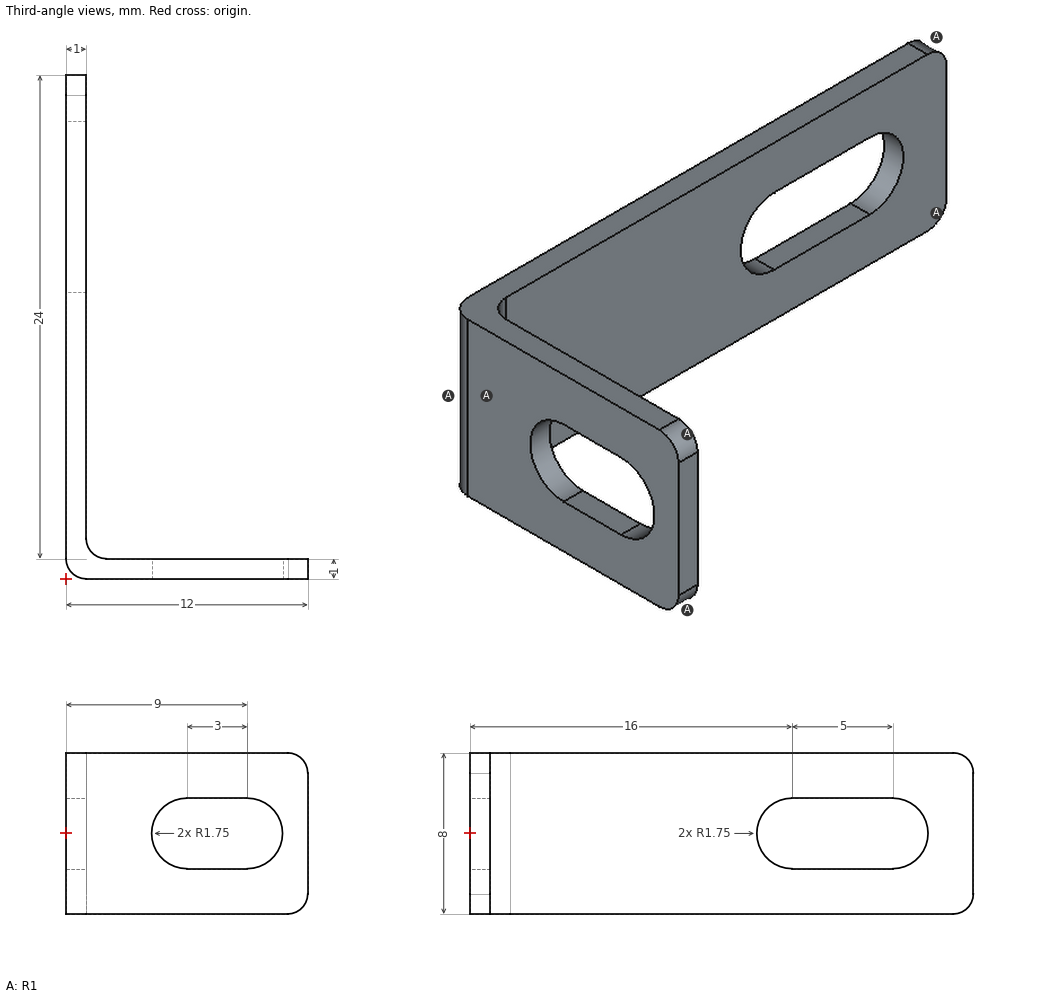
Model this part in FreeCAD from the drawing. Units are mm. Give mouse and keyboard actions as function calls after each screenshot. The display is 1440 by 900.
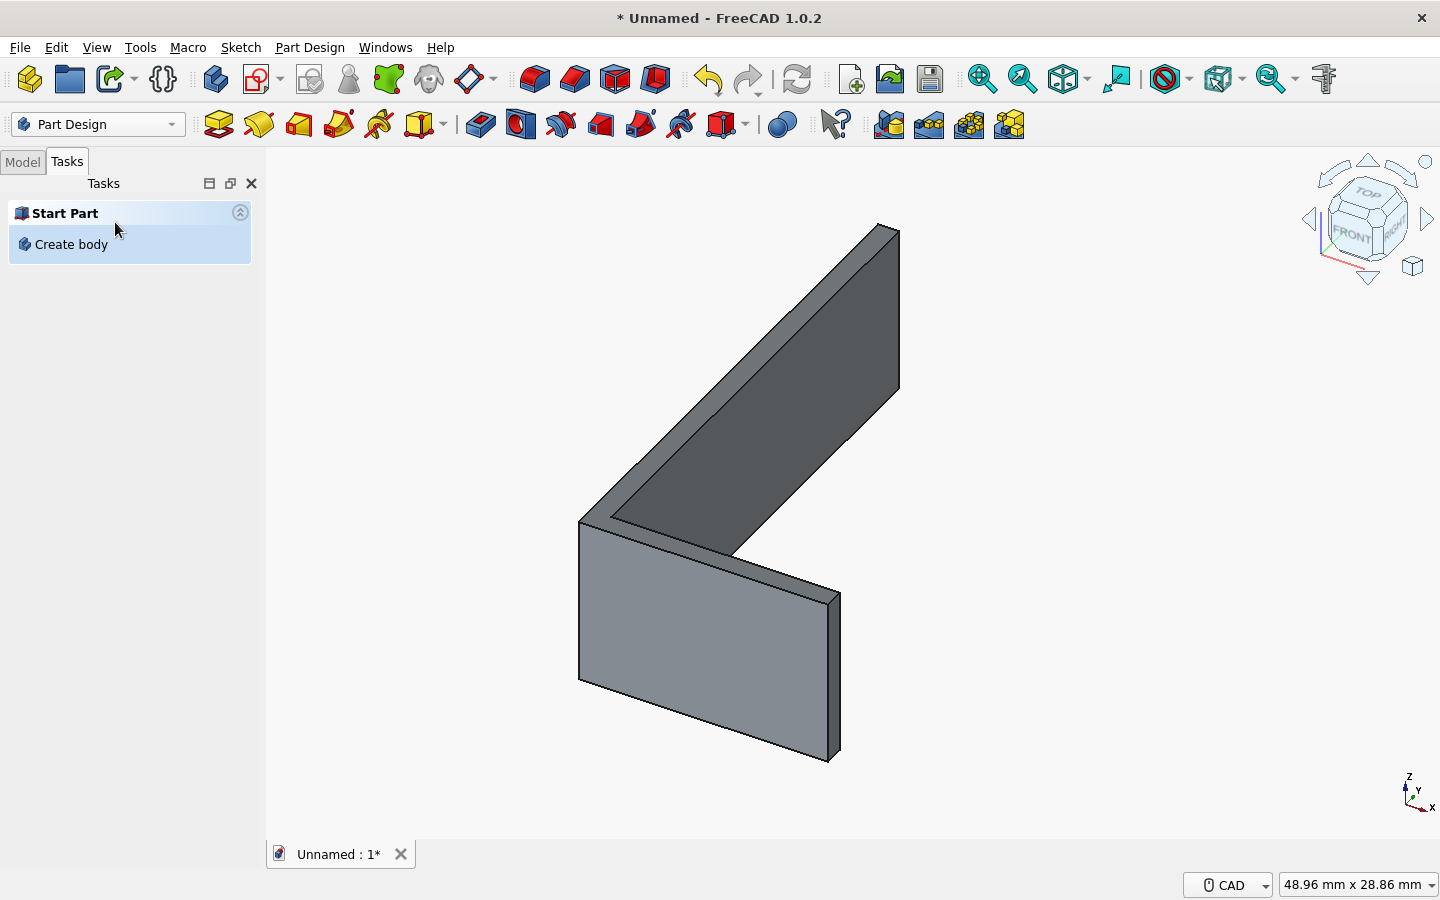
key(4)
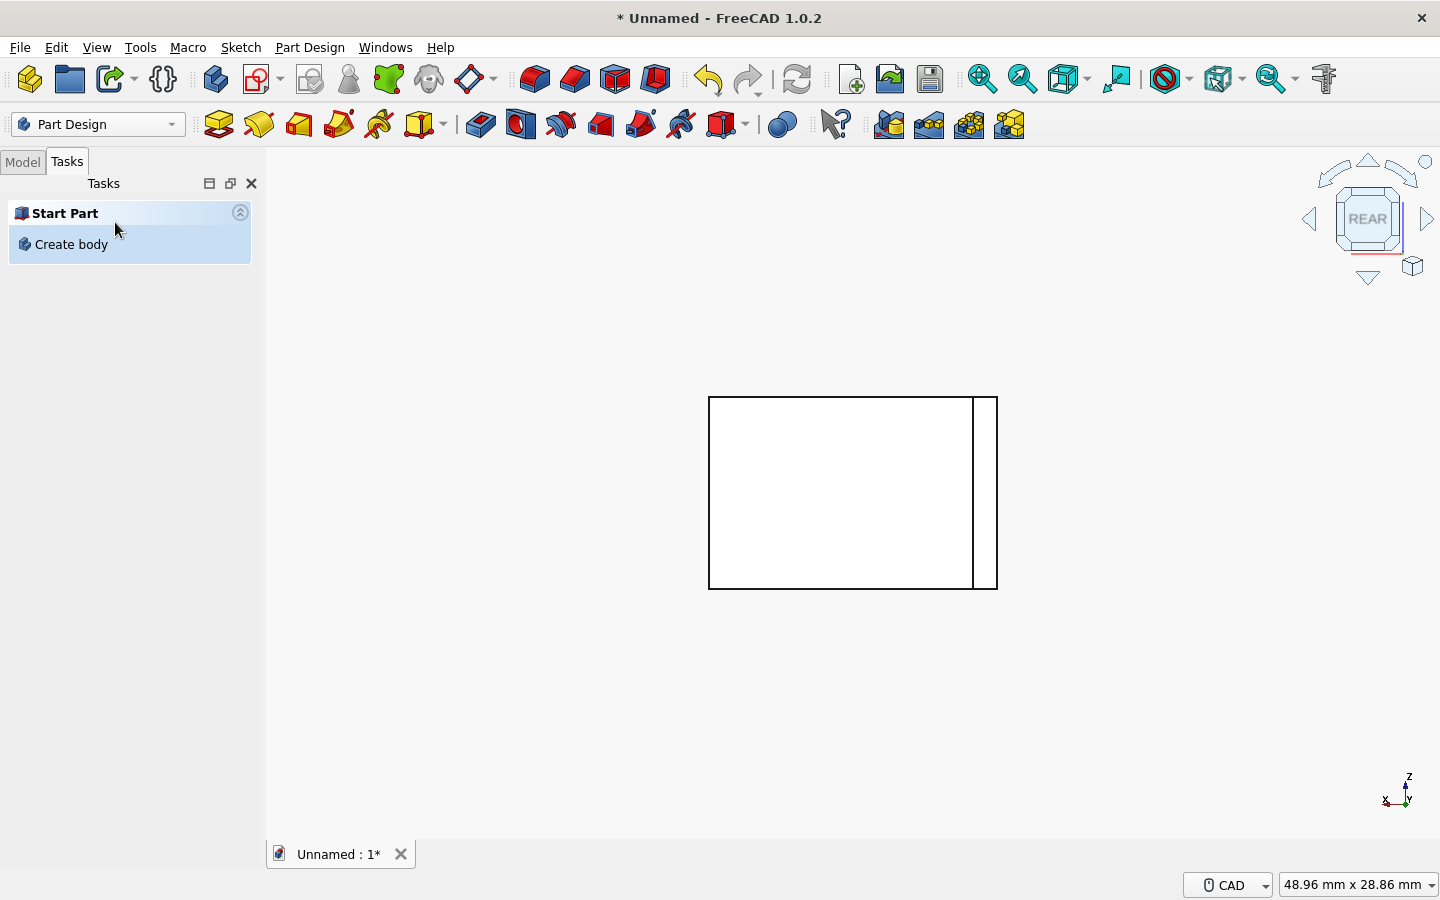
key(v)
key(f)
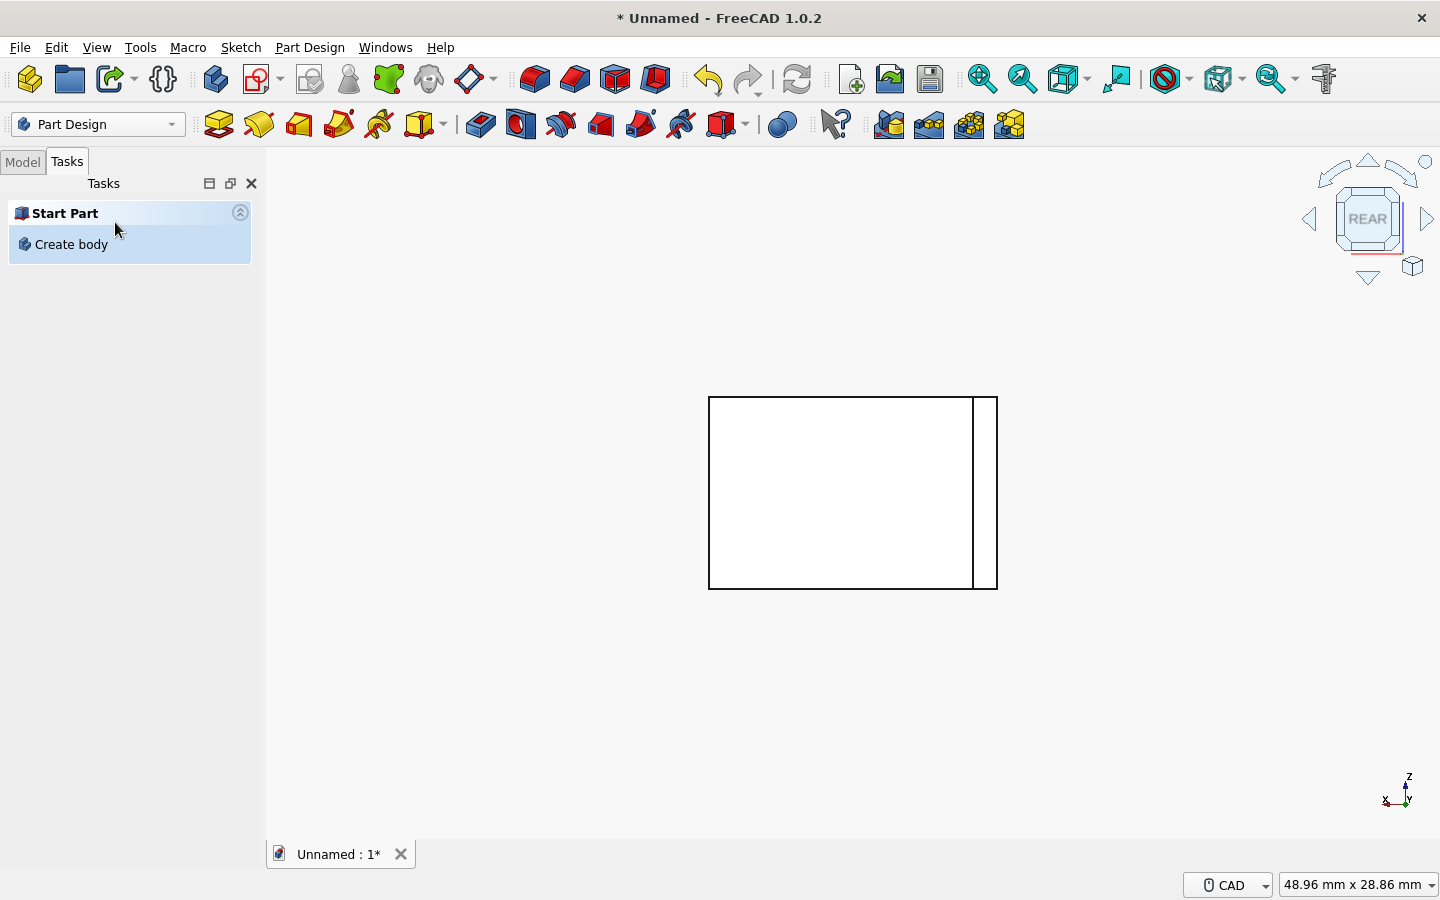
click(841, 492)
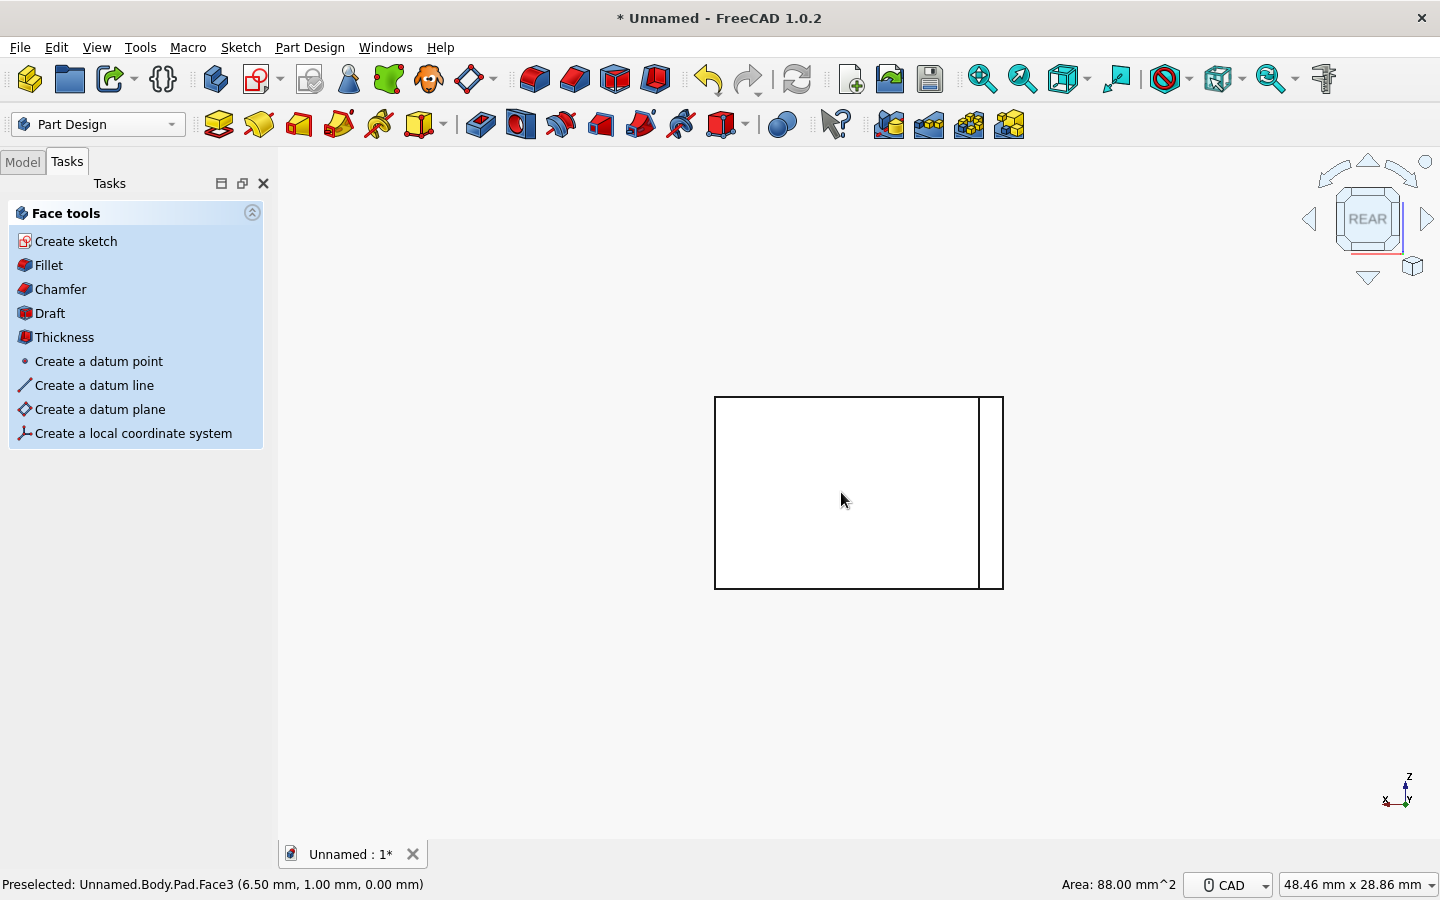
click(256, 80)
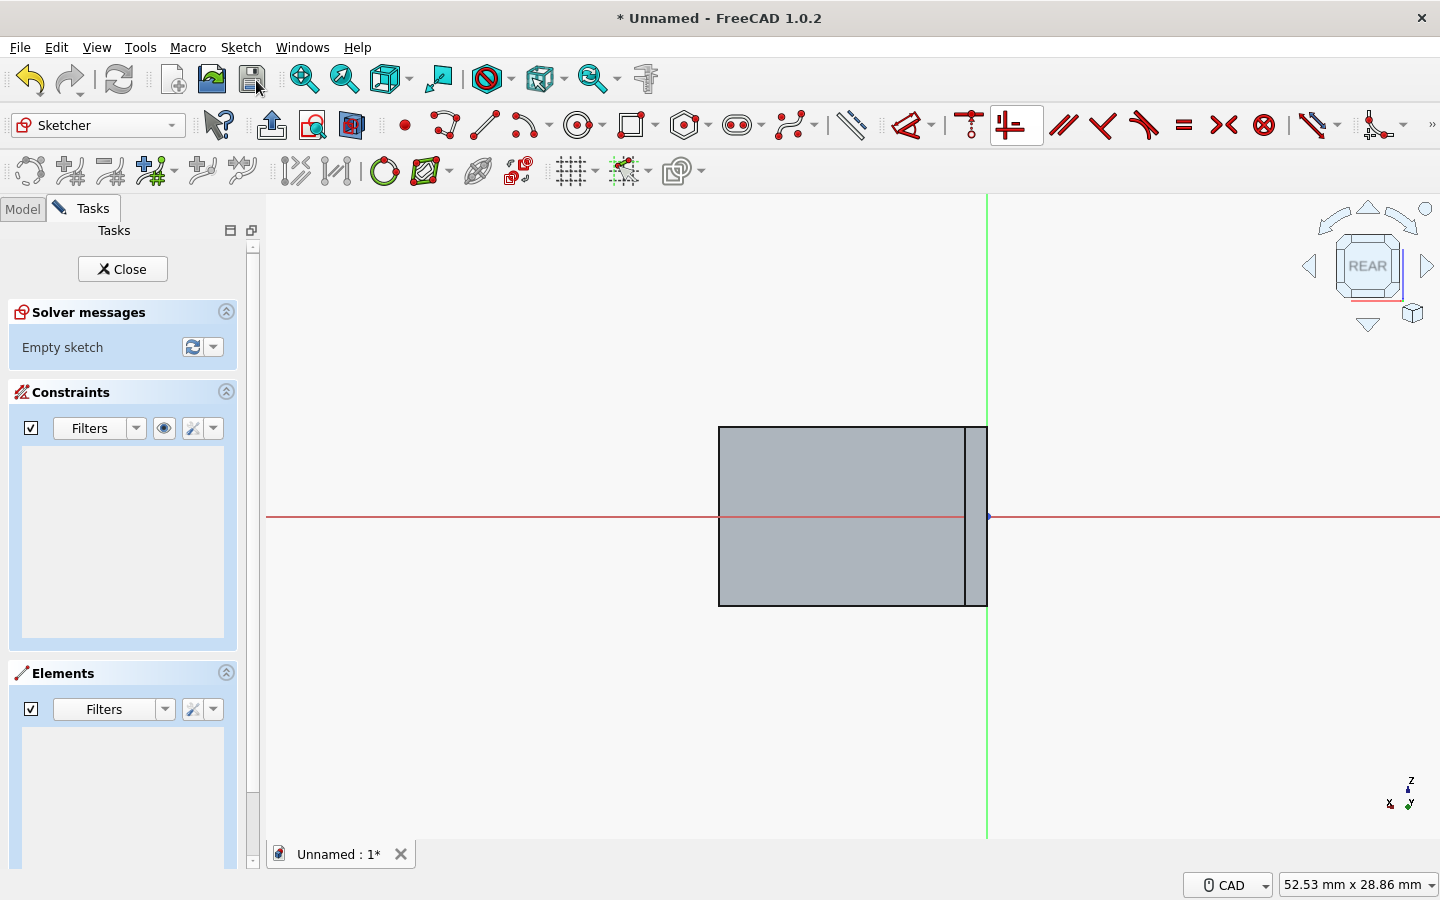
scroll(915, 517, up, 5)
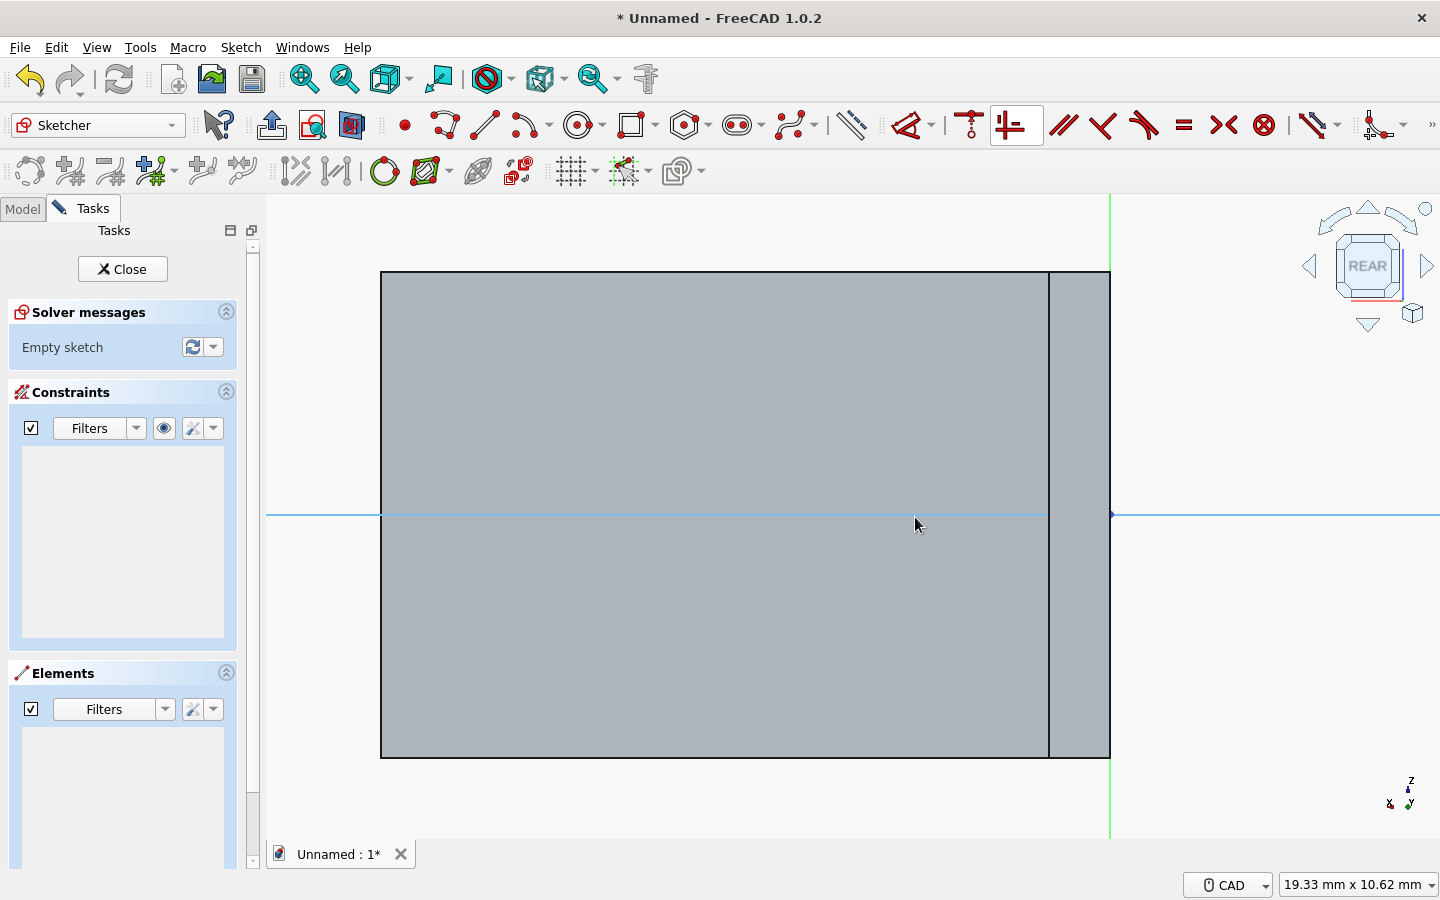
key(g)
key(s)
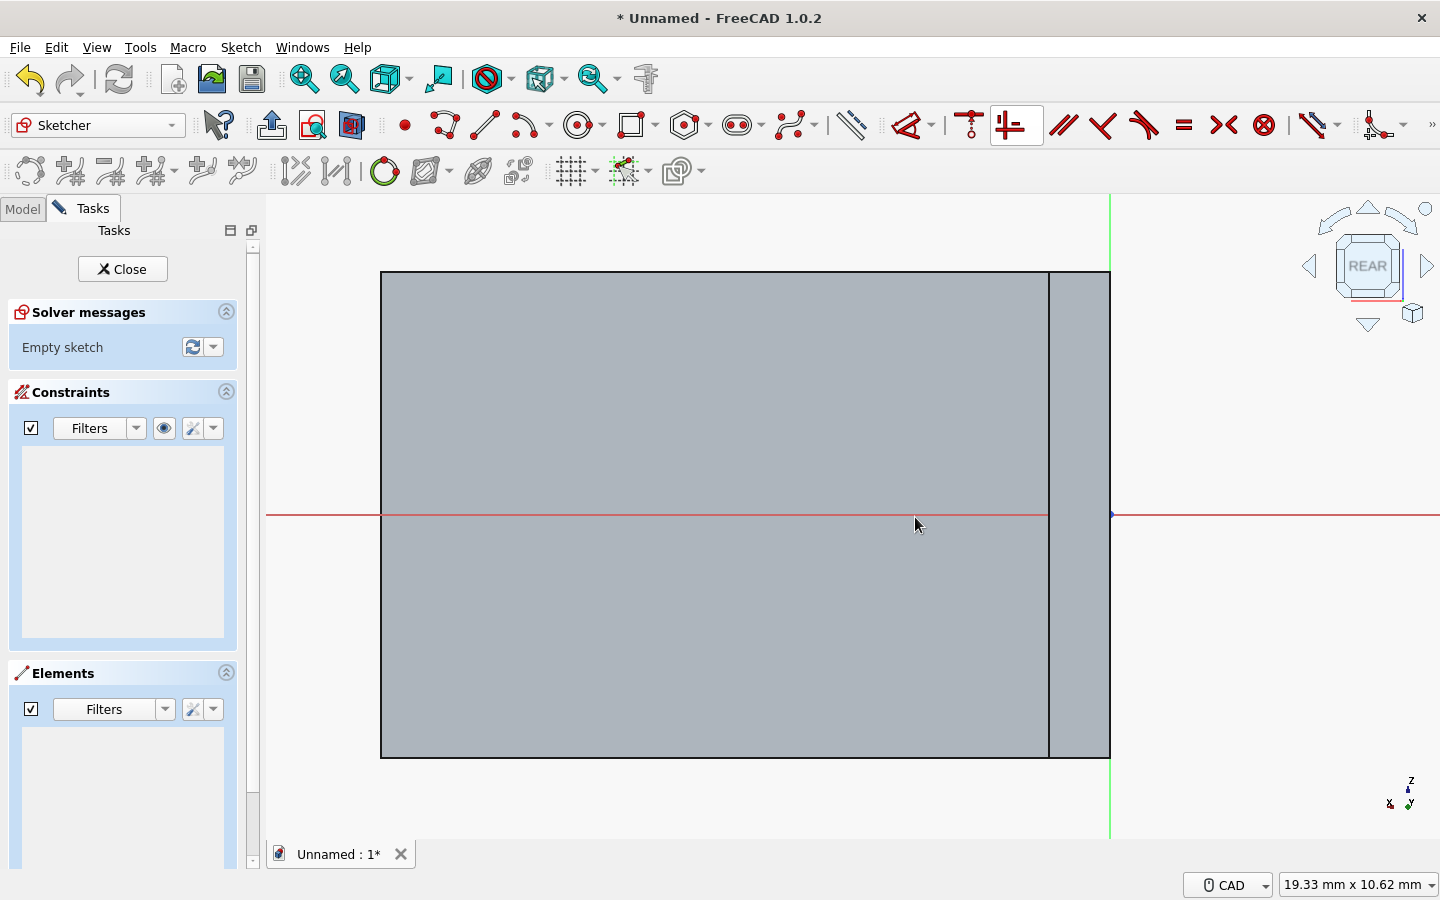
click(563, 515)